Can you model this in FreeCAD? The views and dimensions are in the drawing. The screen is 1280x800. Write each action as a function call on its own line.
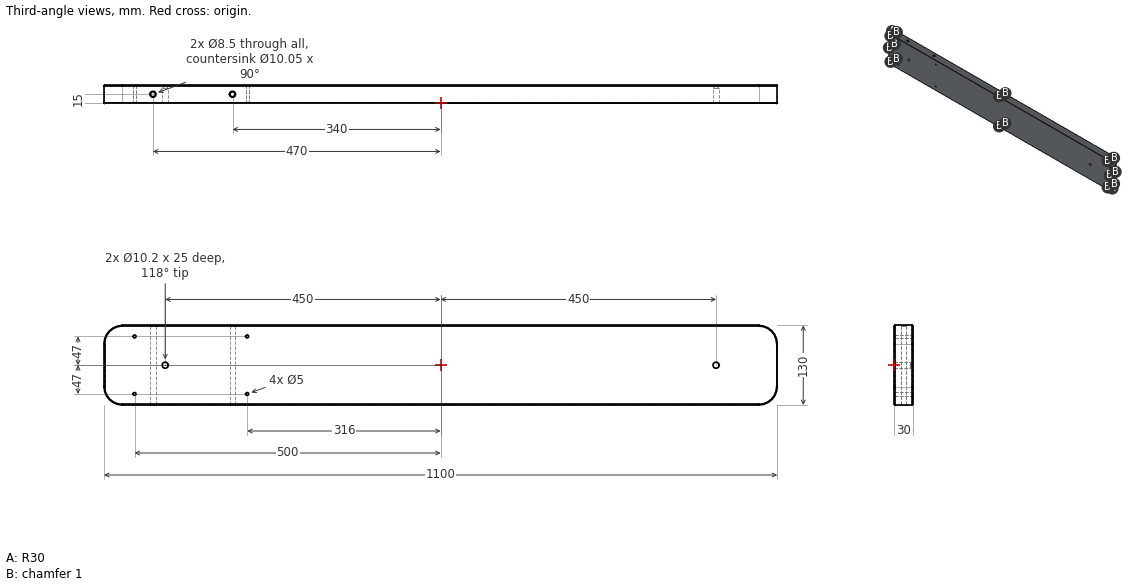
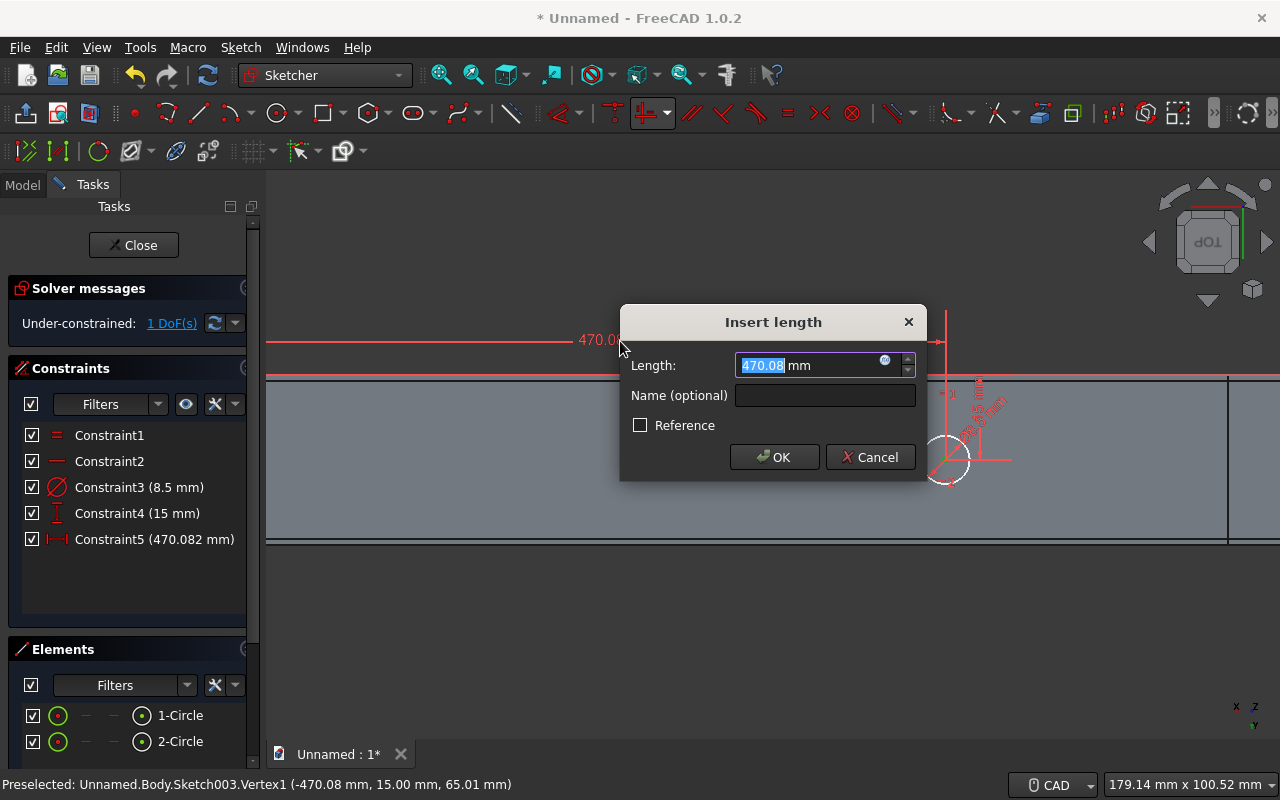
text(470)
key(Return)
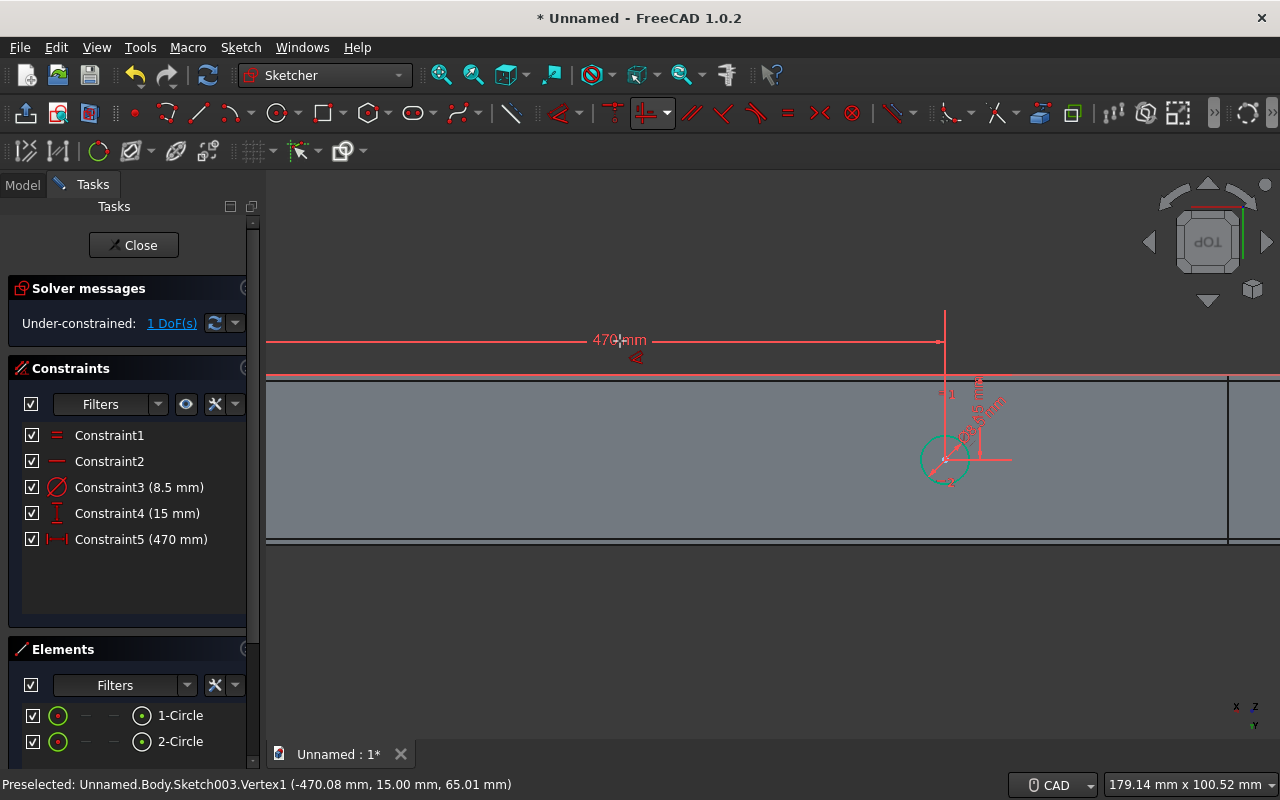
scroll(963, 443, down, 2)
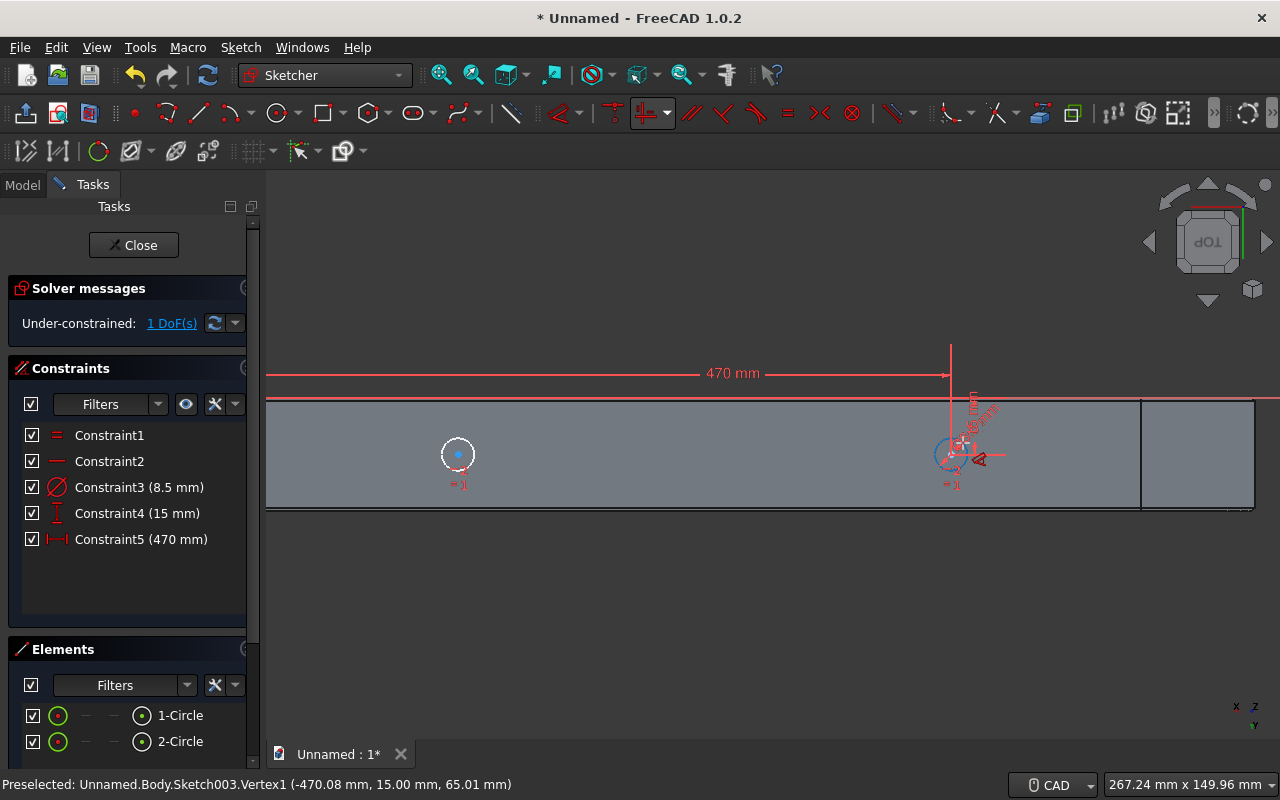
click(458, 454)
click(376, 364)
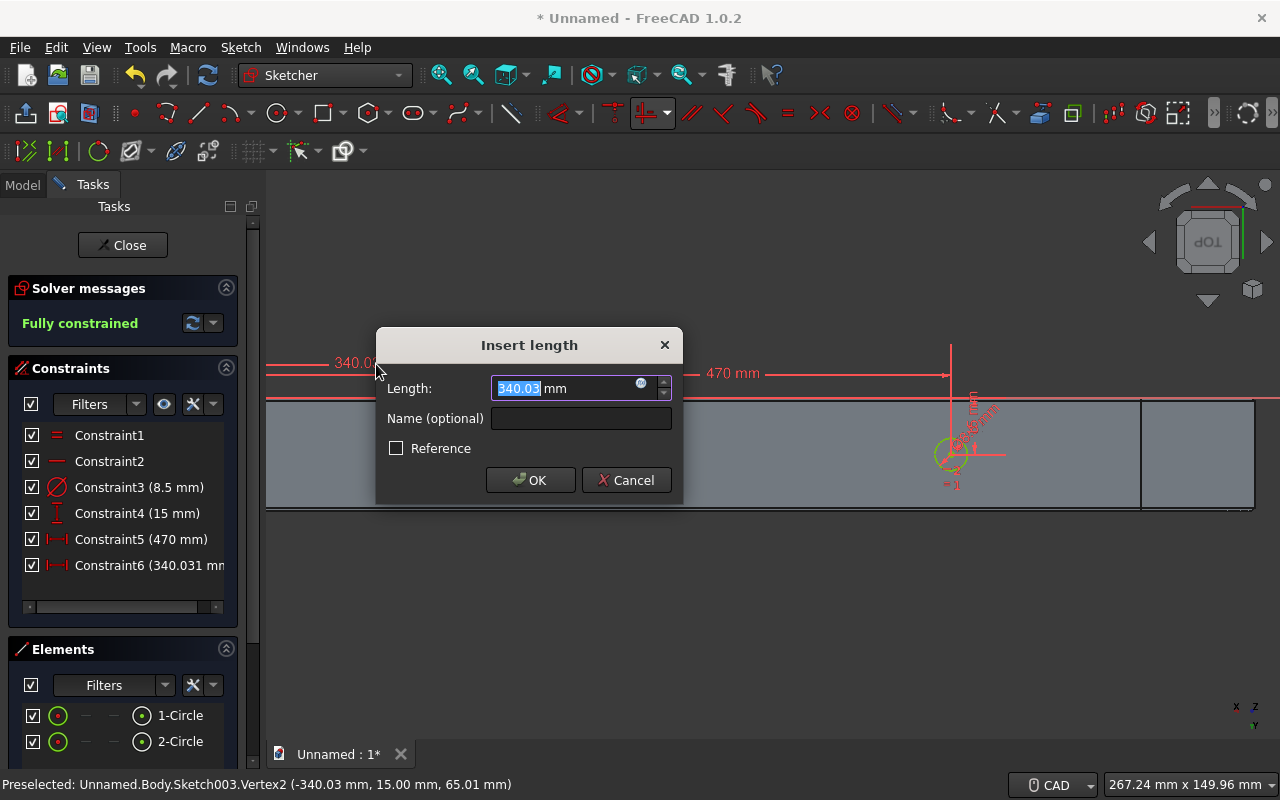
text(340)
key(Return)
key(Escape)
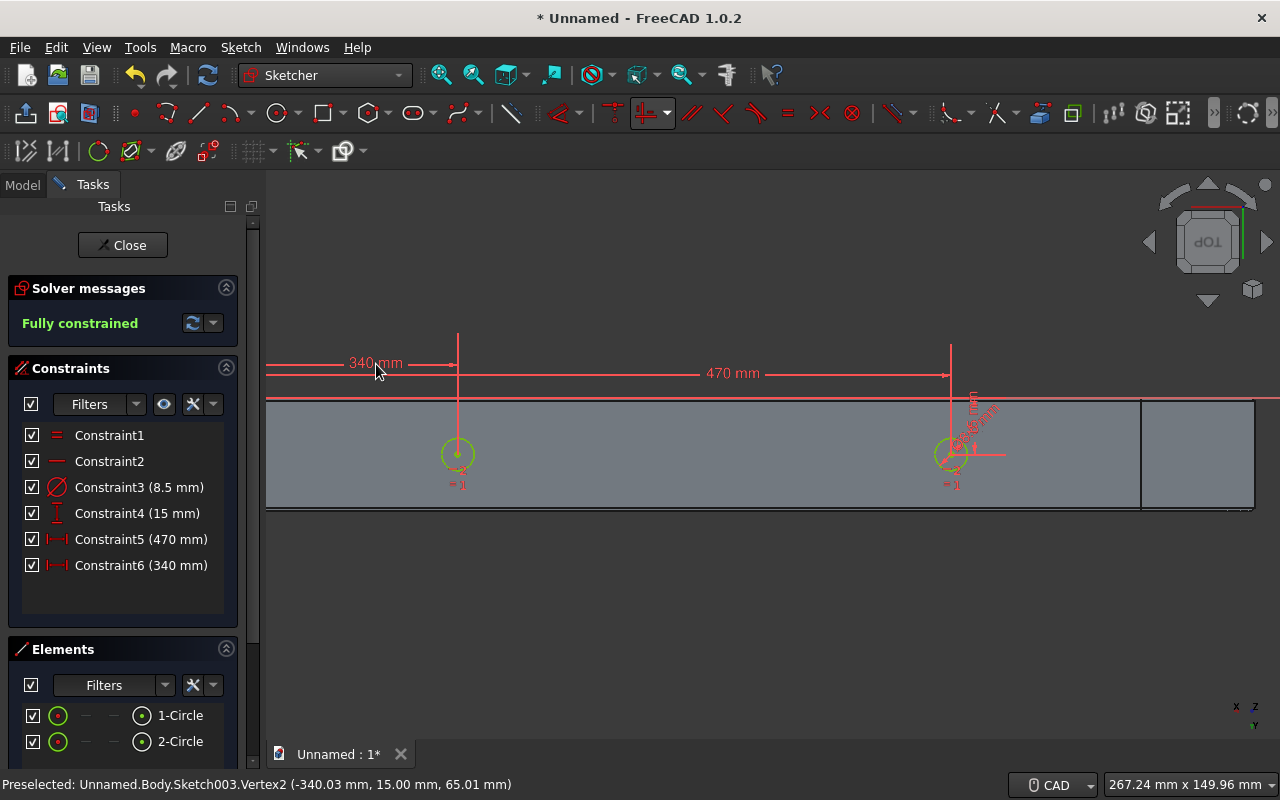
click(123, 245)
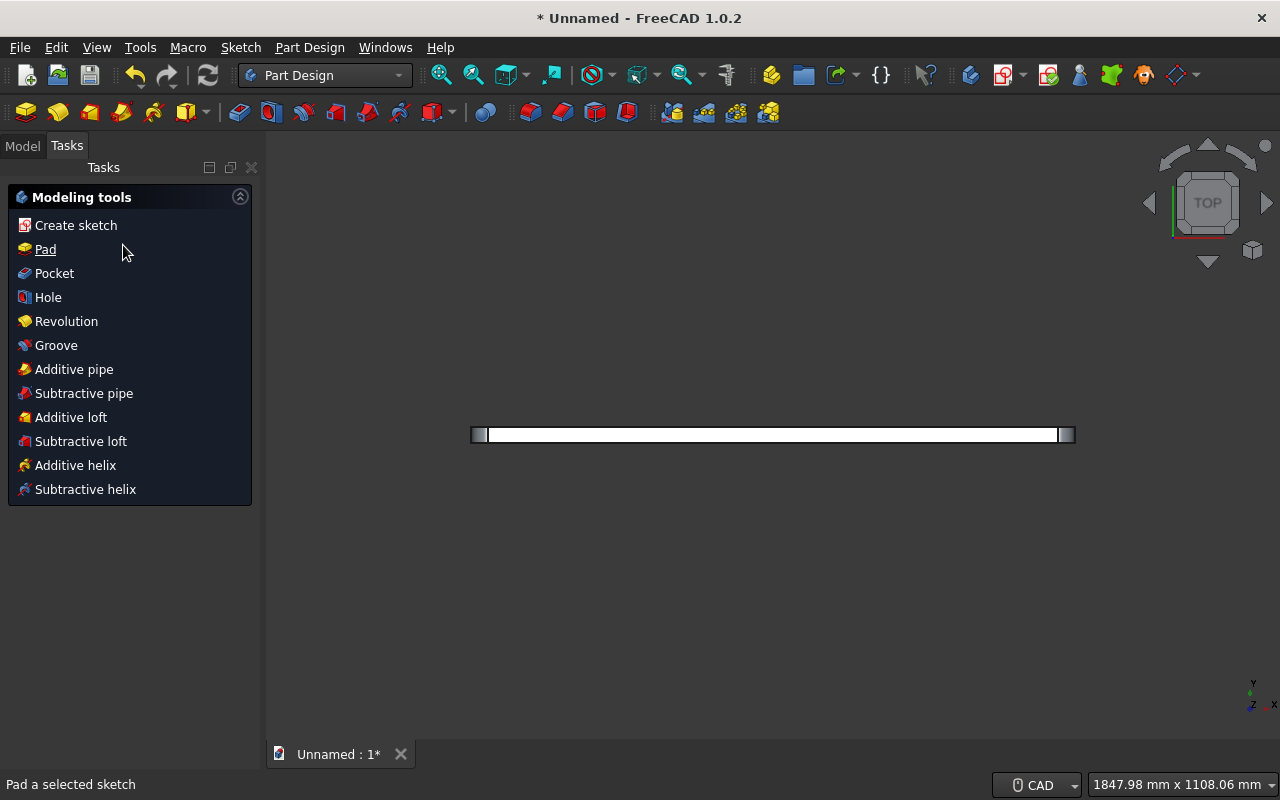
click(272, 112)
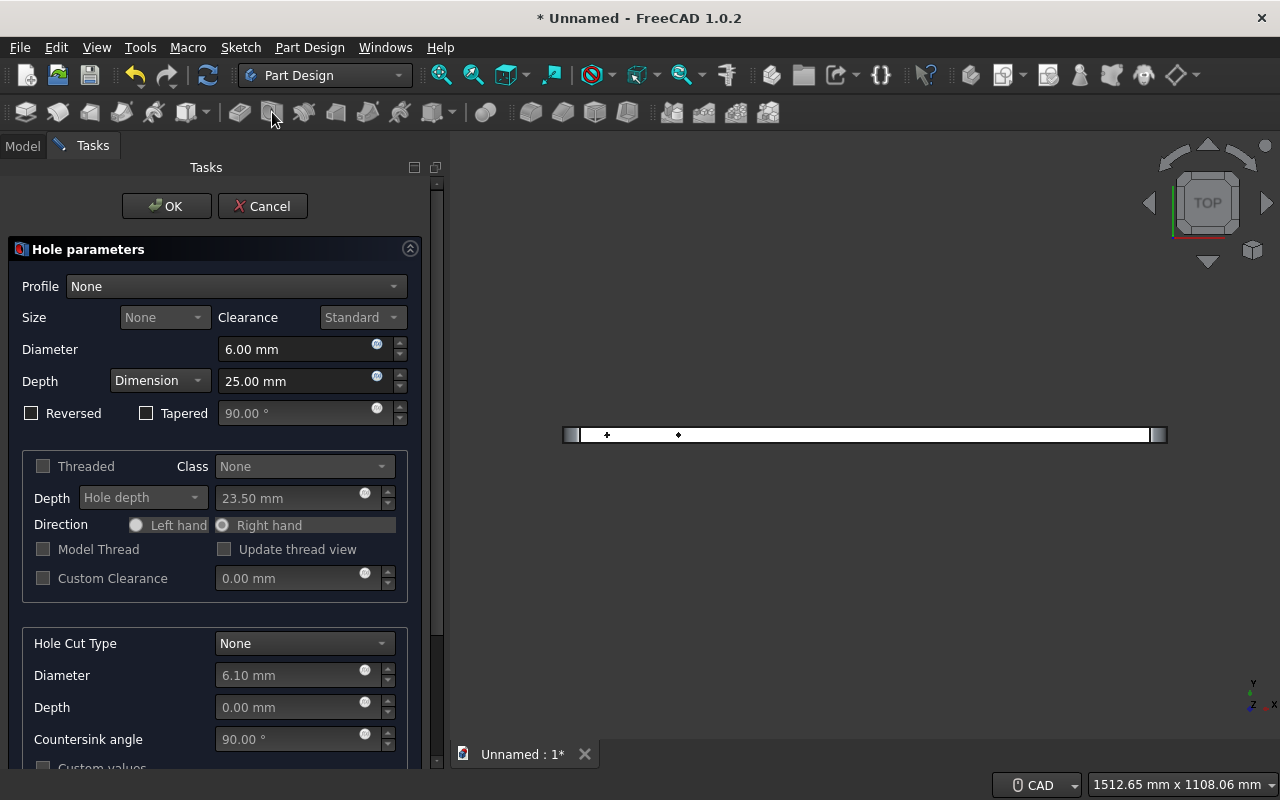
triple_click(305, 349)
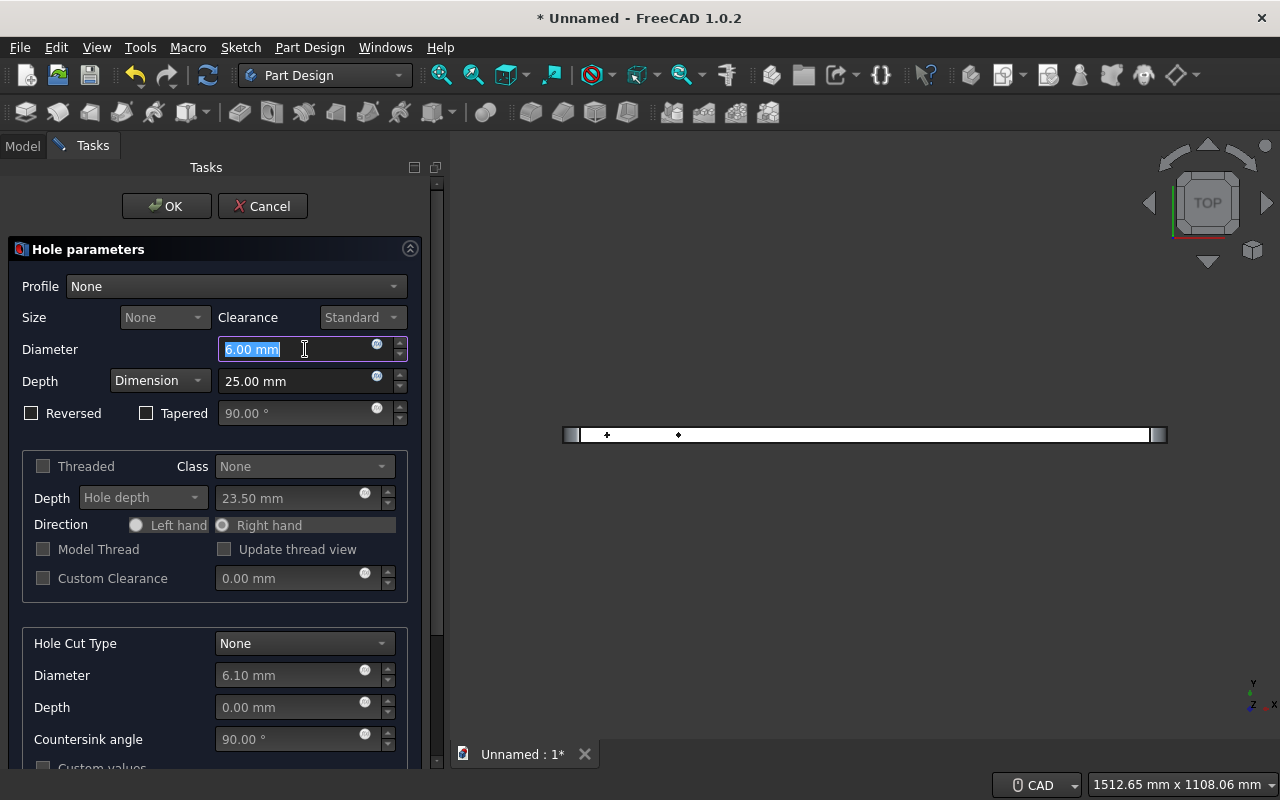
text(8.5)
key(Tab)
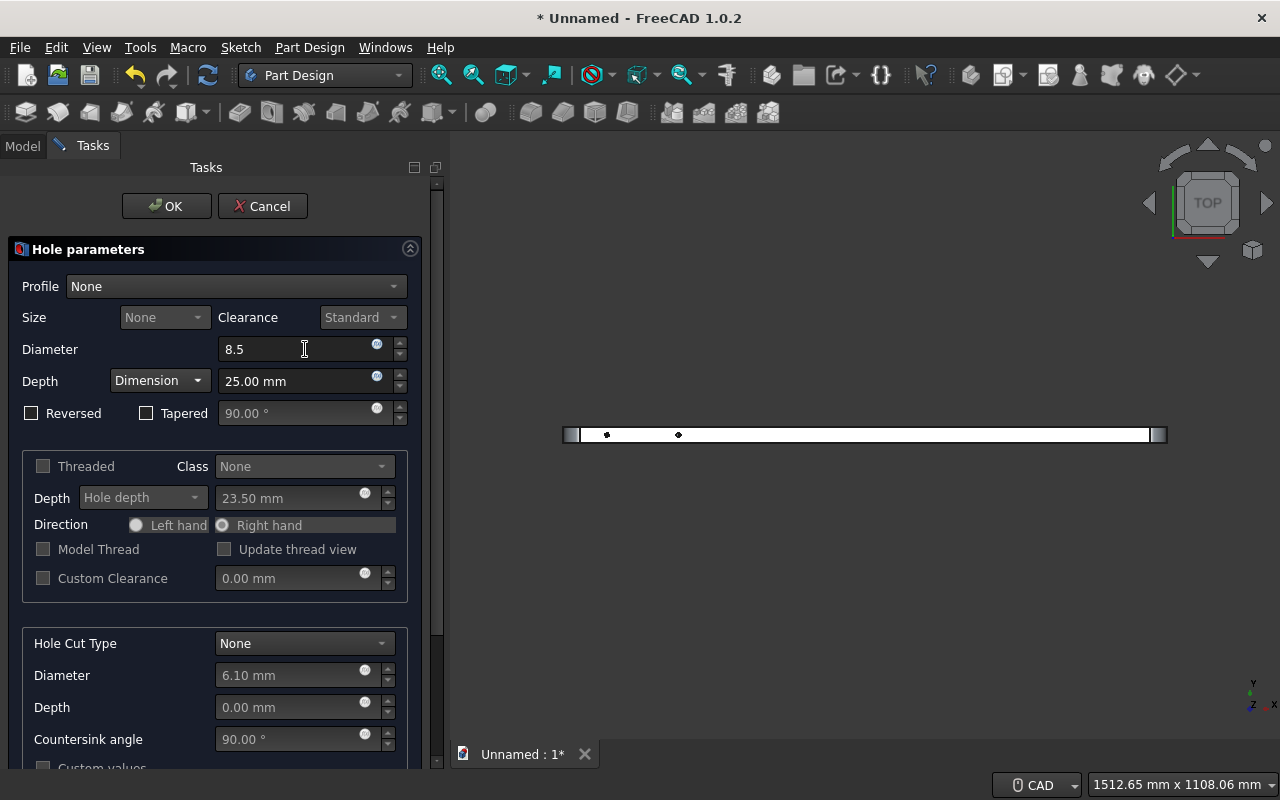
click(161, 380)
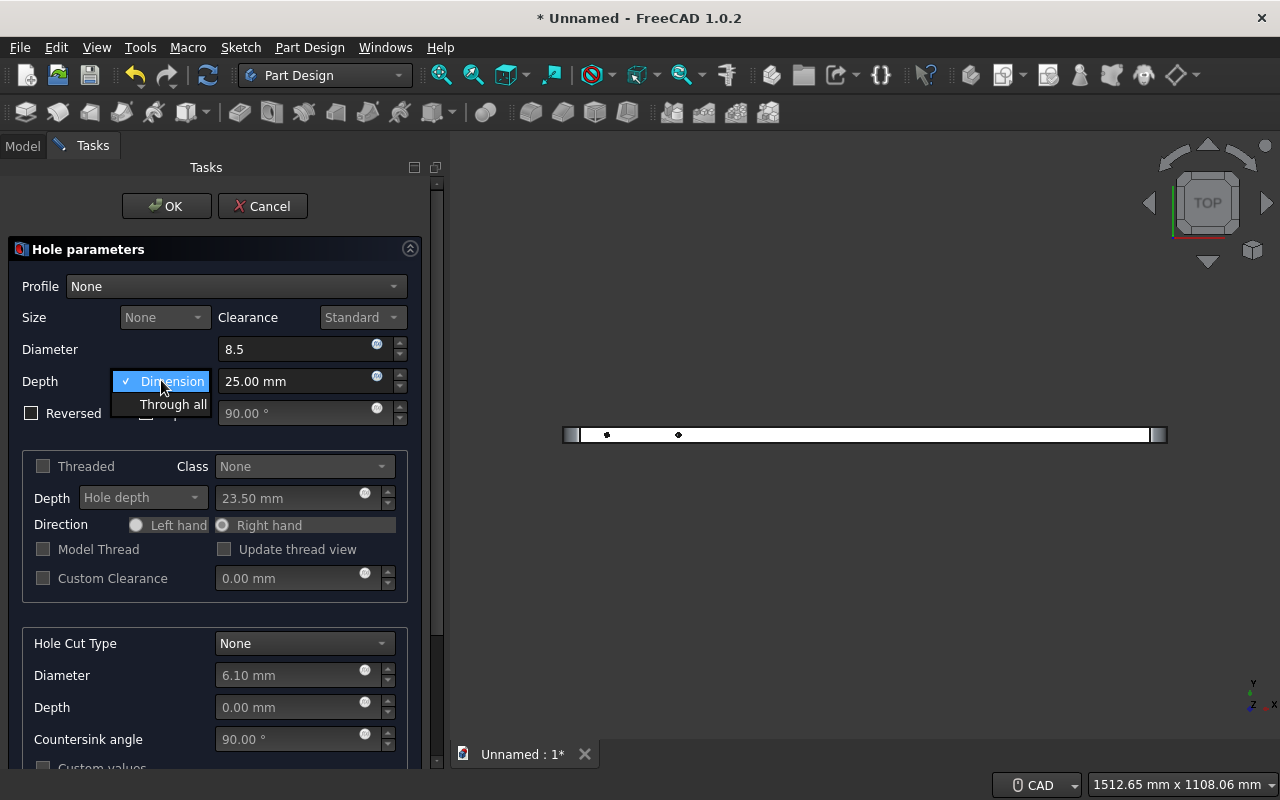
click(160, 404)